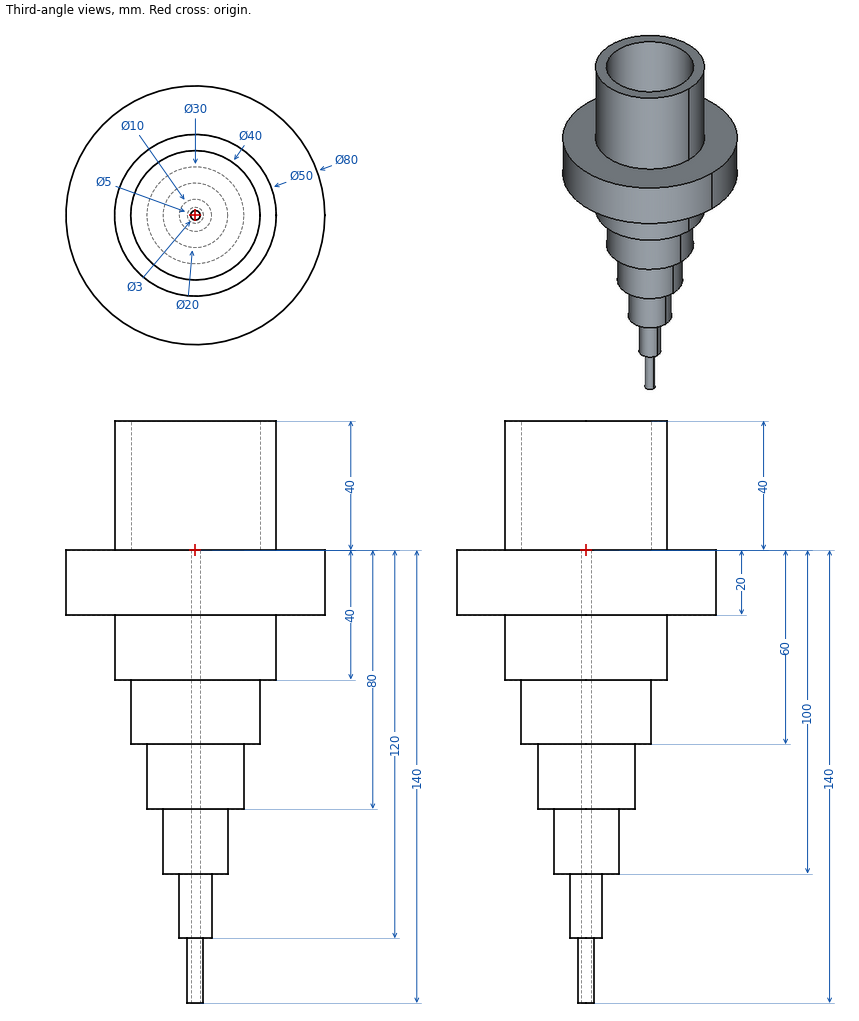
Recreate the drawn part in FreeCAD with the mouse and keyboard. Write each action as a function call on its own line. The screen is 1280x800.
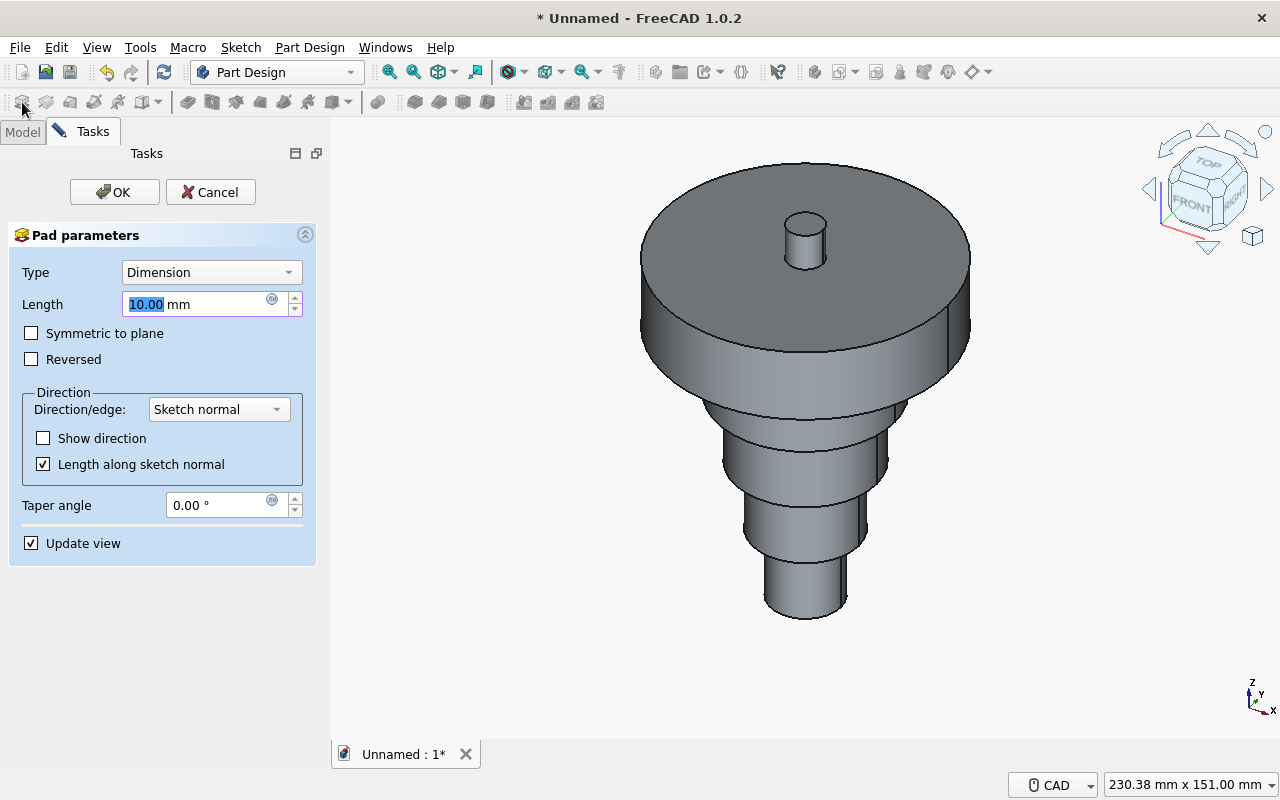
text(120)
key(Tab)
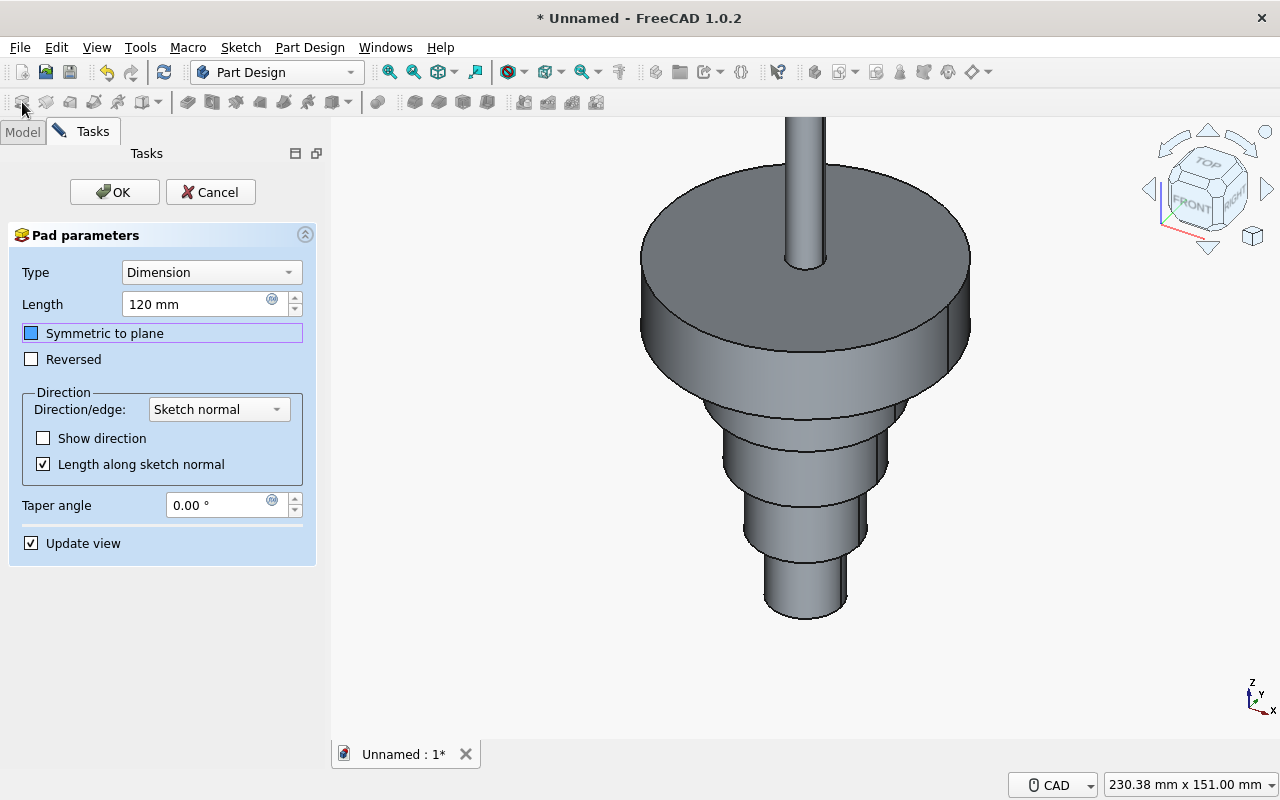
click(30, 359)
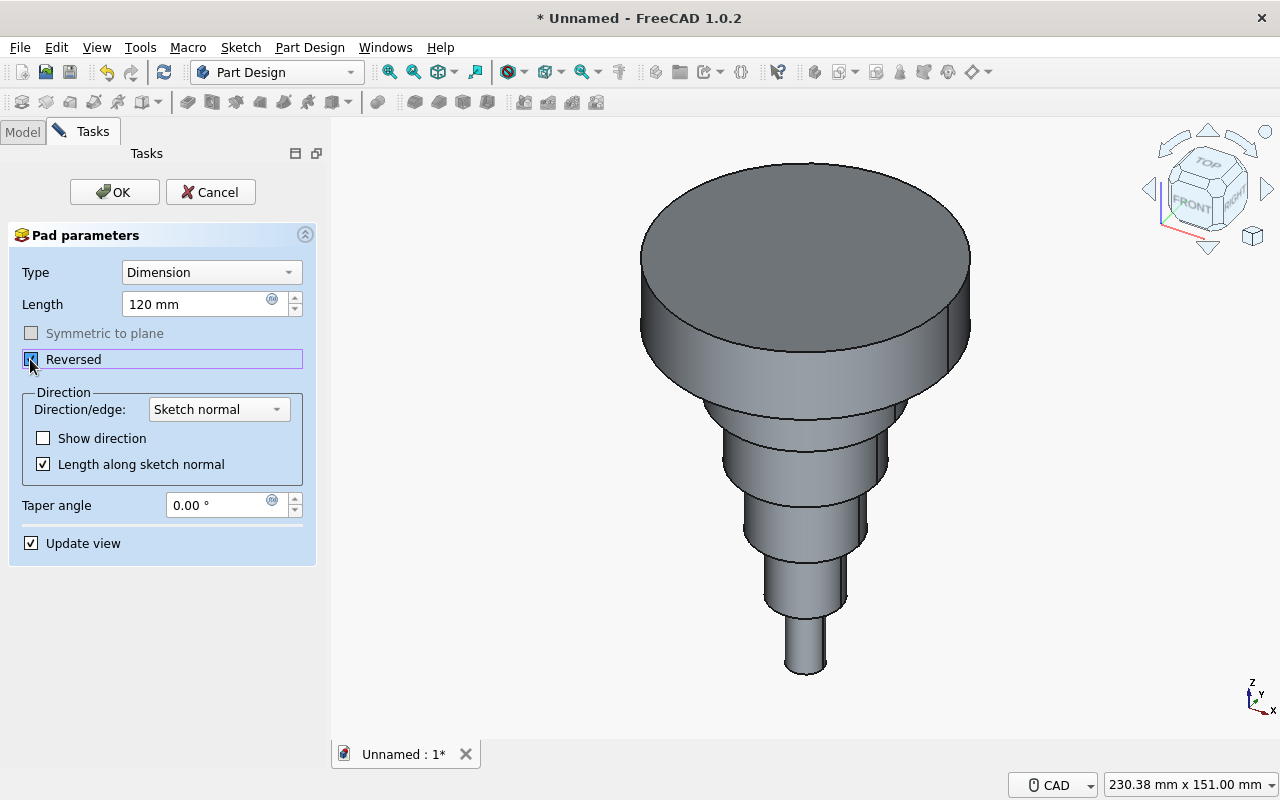
click(115, 192)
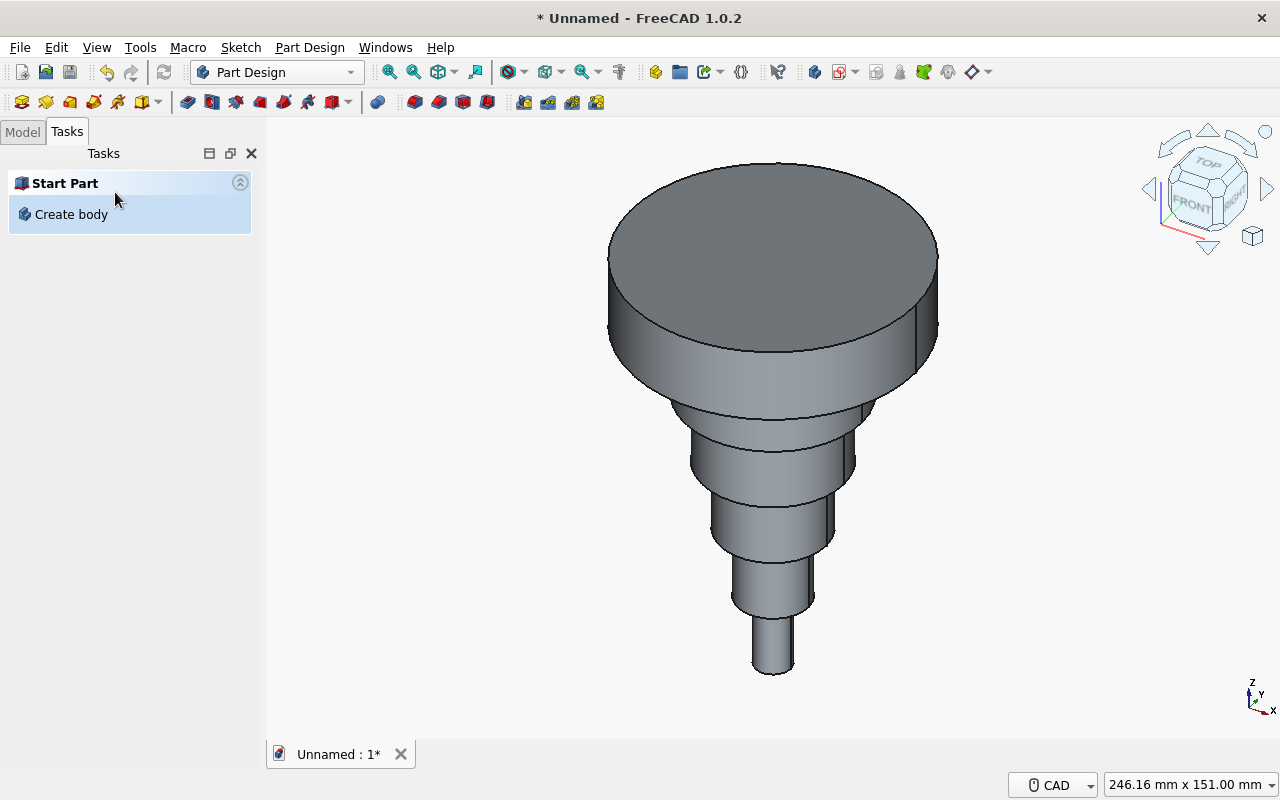
key(v)
key(f)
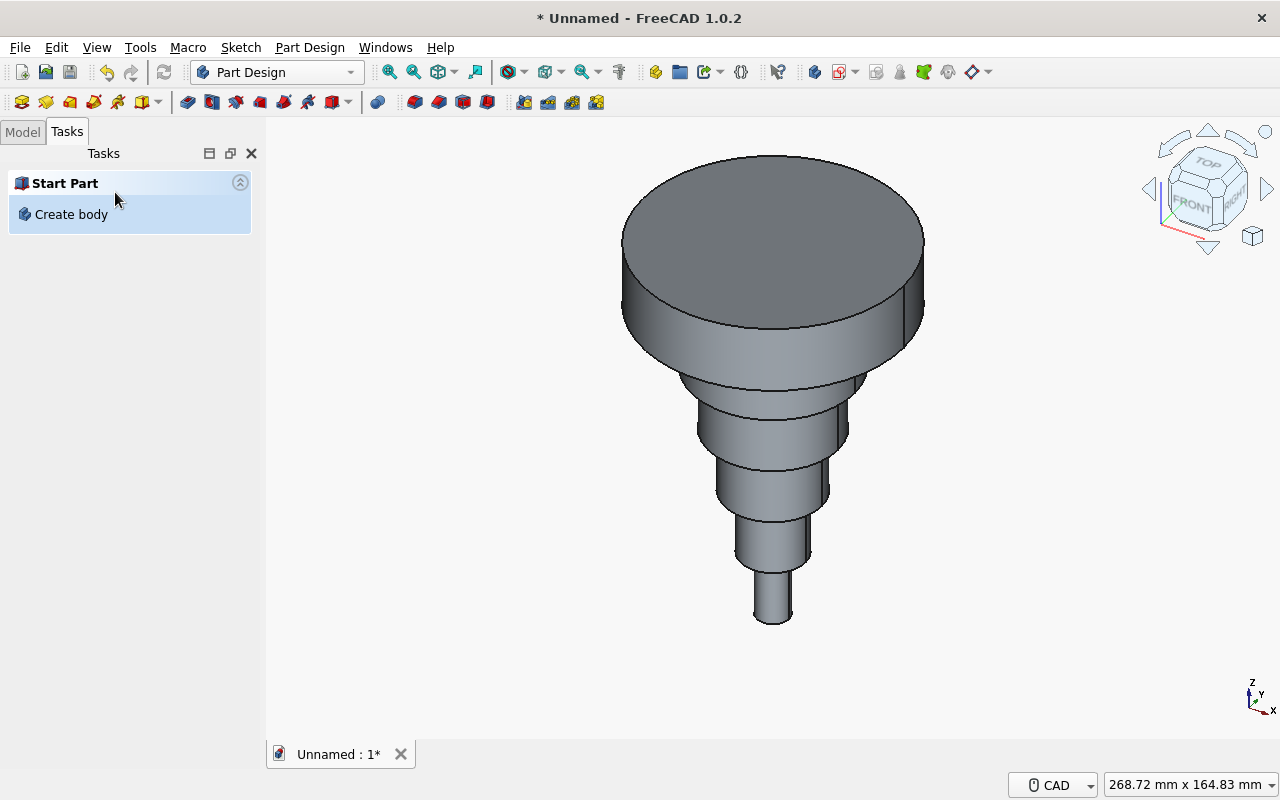
click(773, 242)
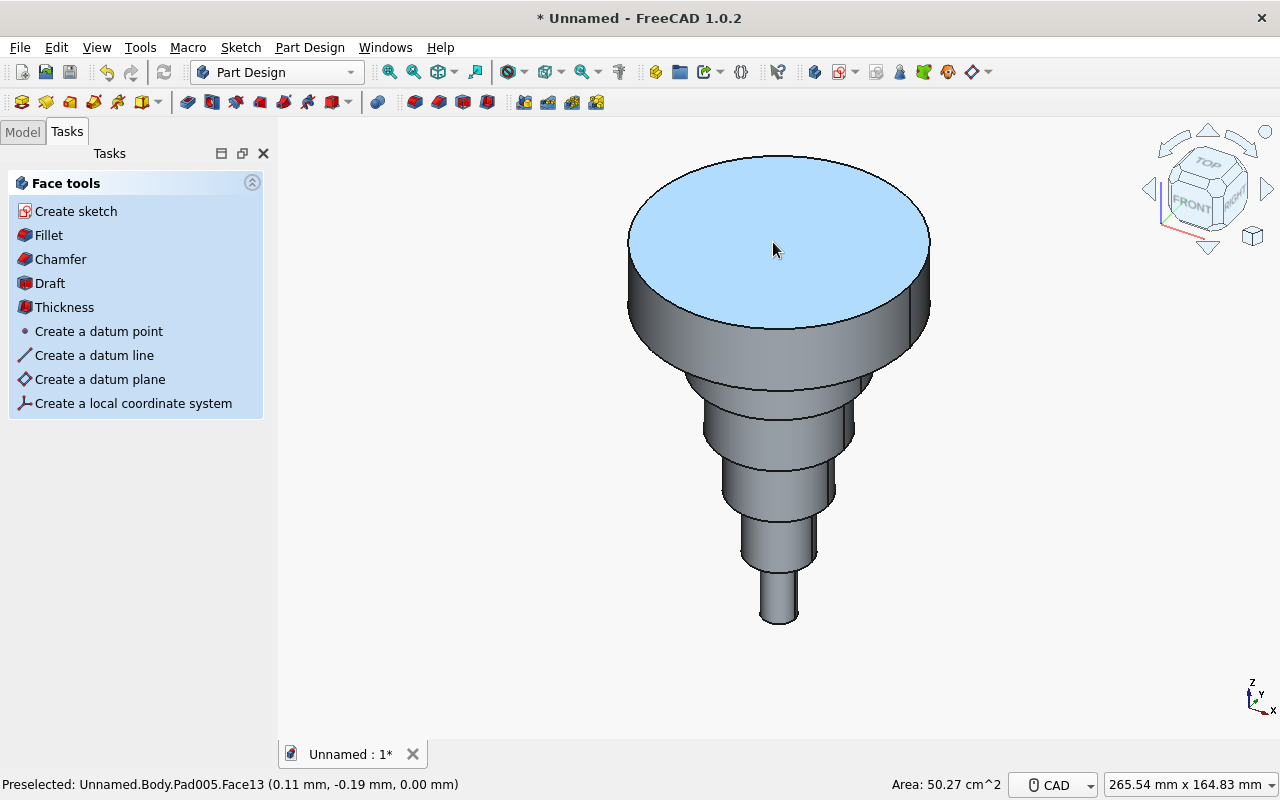
click(840, 72)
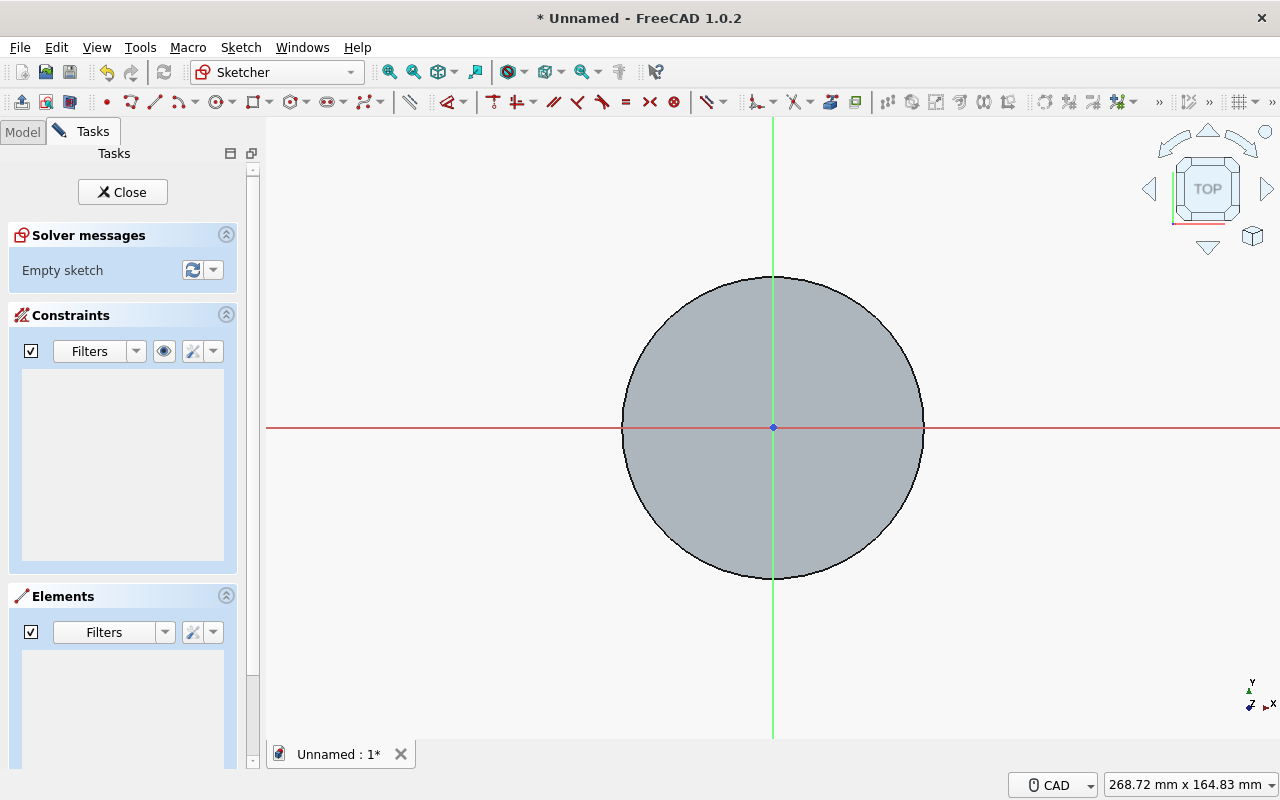
scroll(777, 428, up, 15)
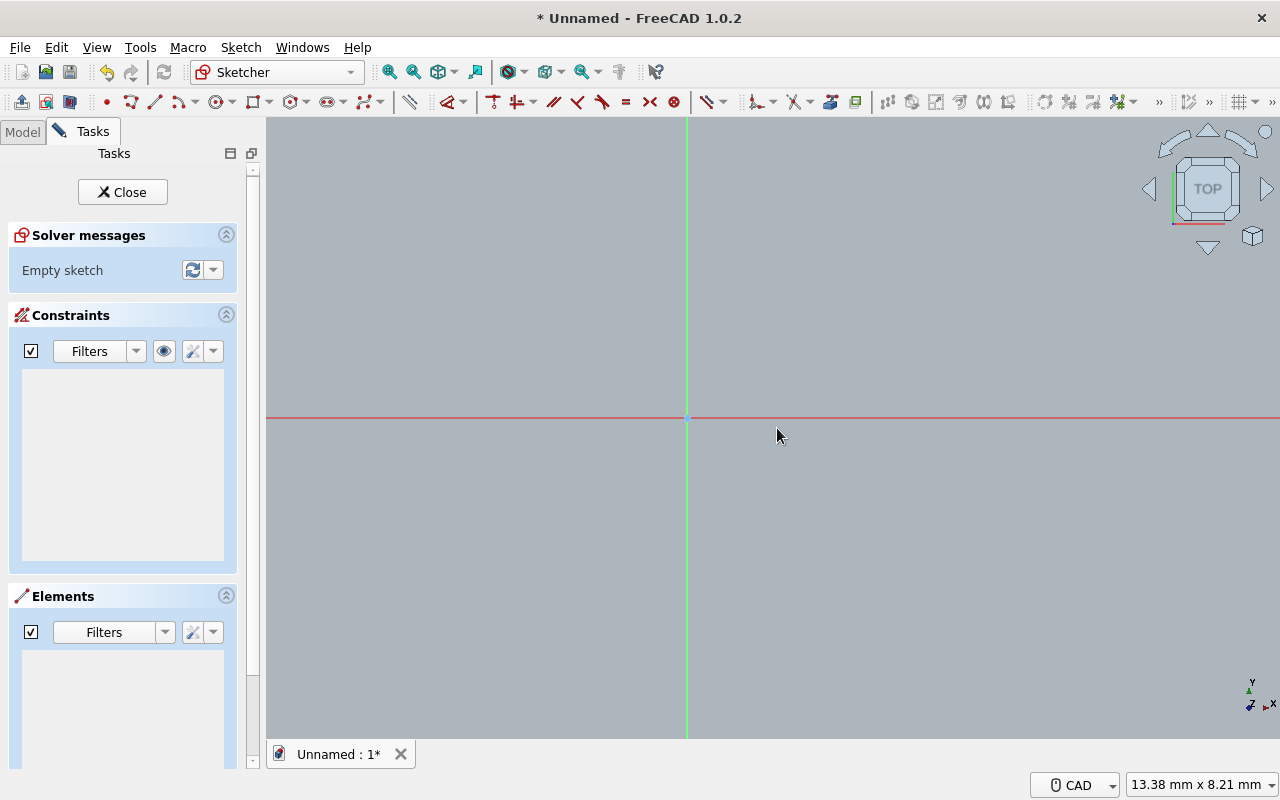
key(g)
key(c)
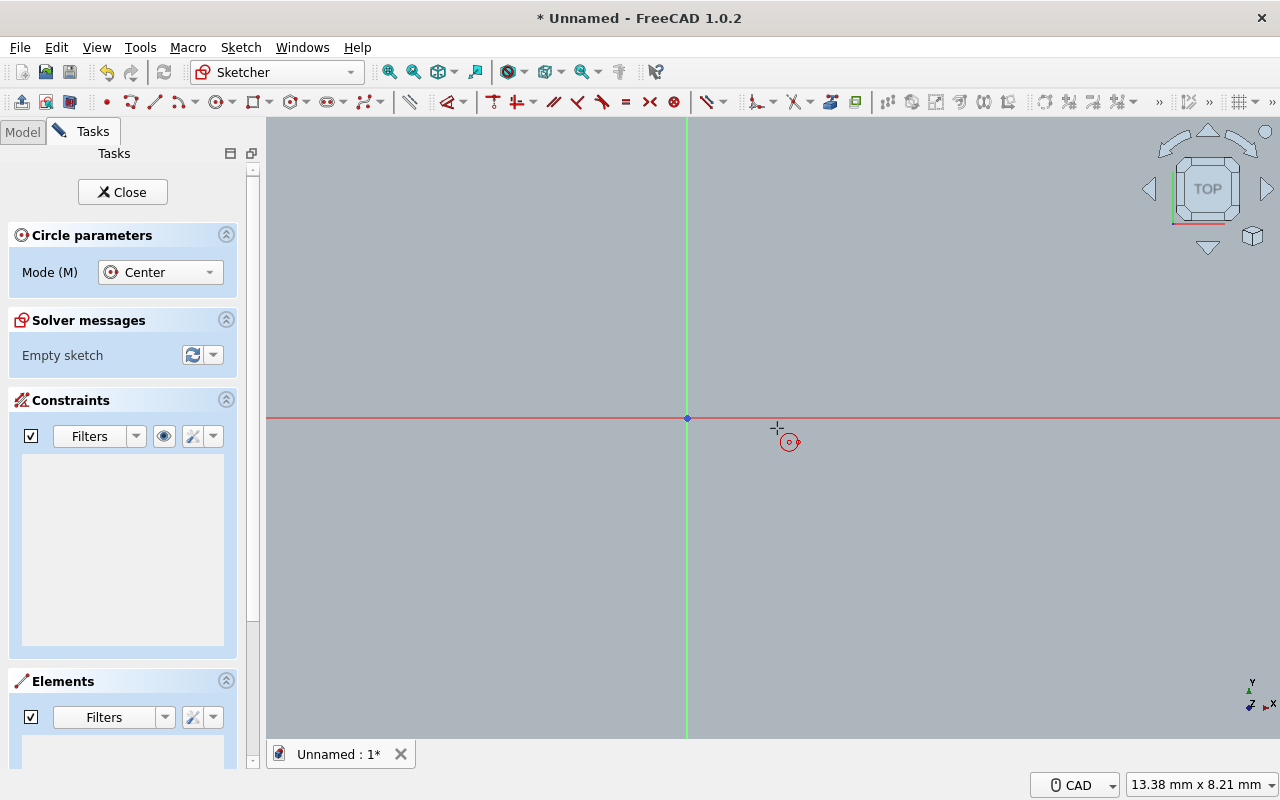
click(687, 418)
move(821, 284)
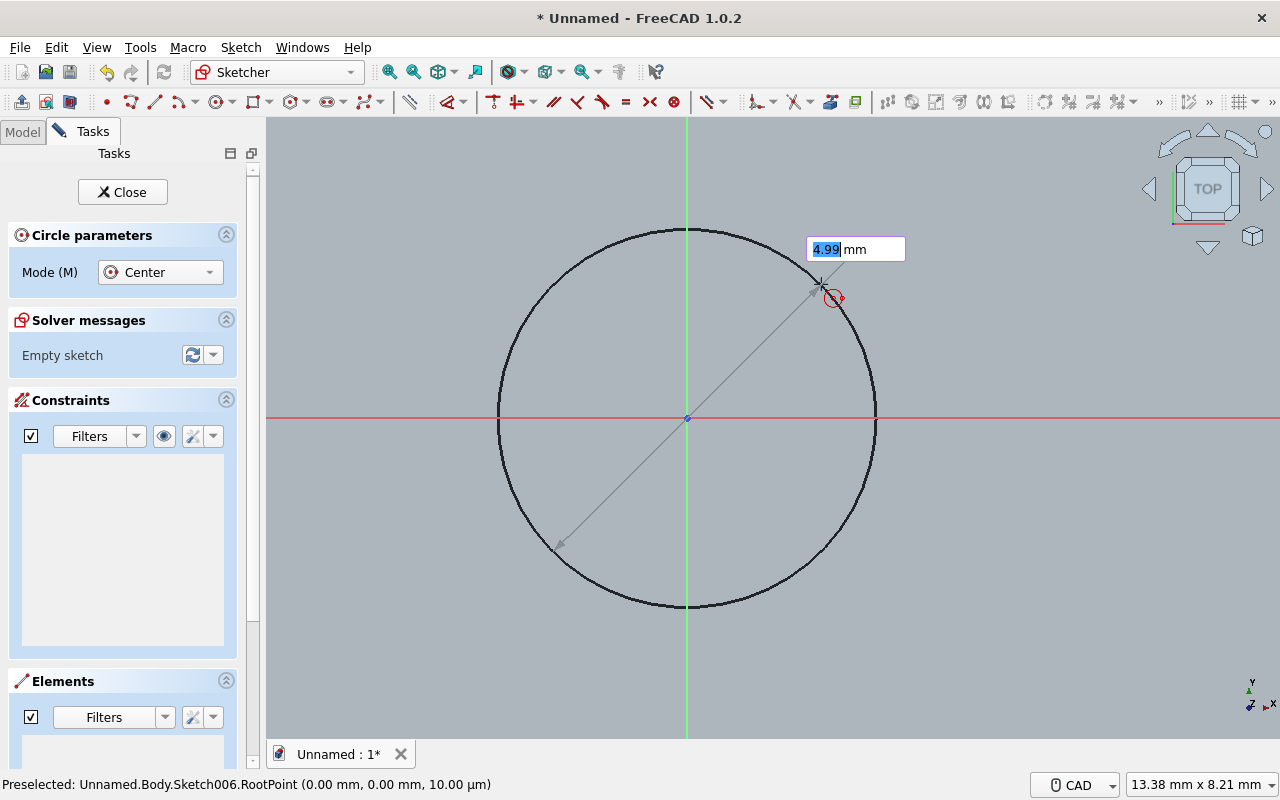
text(5)
key(Return)
key(Escape)